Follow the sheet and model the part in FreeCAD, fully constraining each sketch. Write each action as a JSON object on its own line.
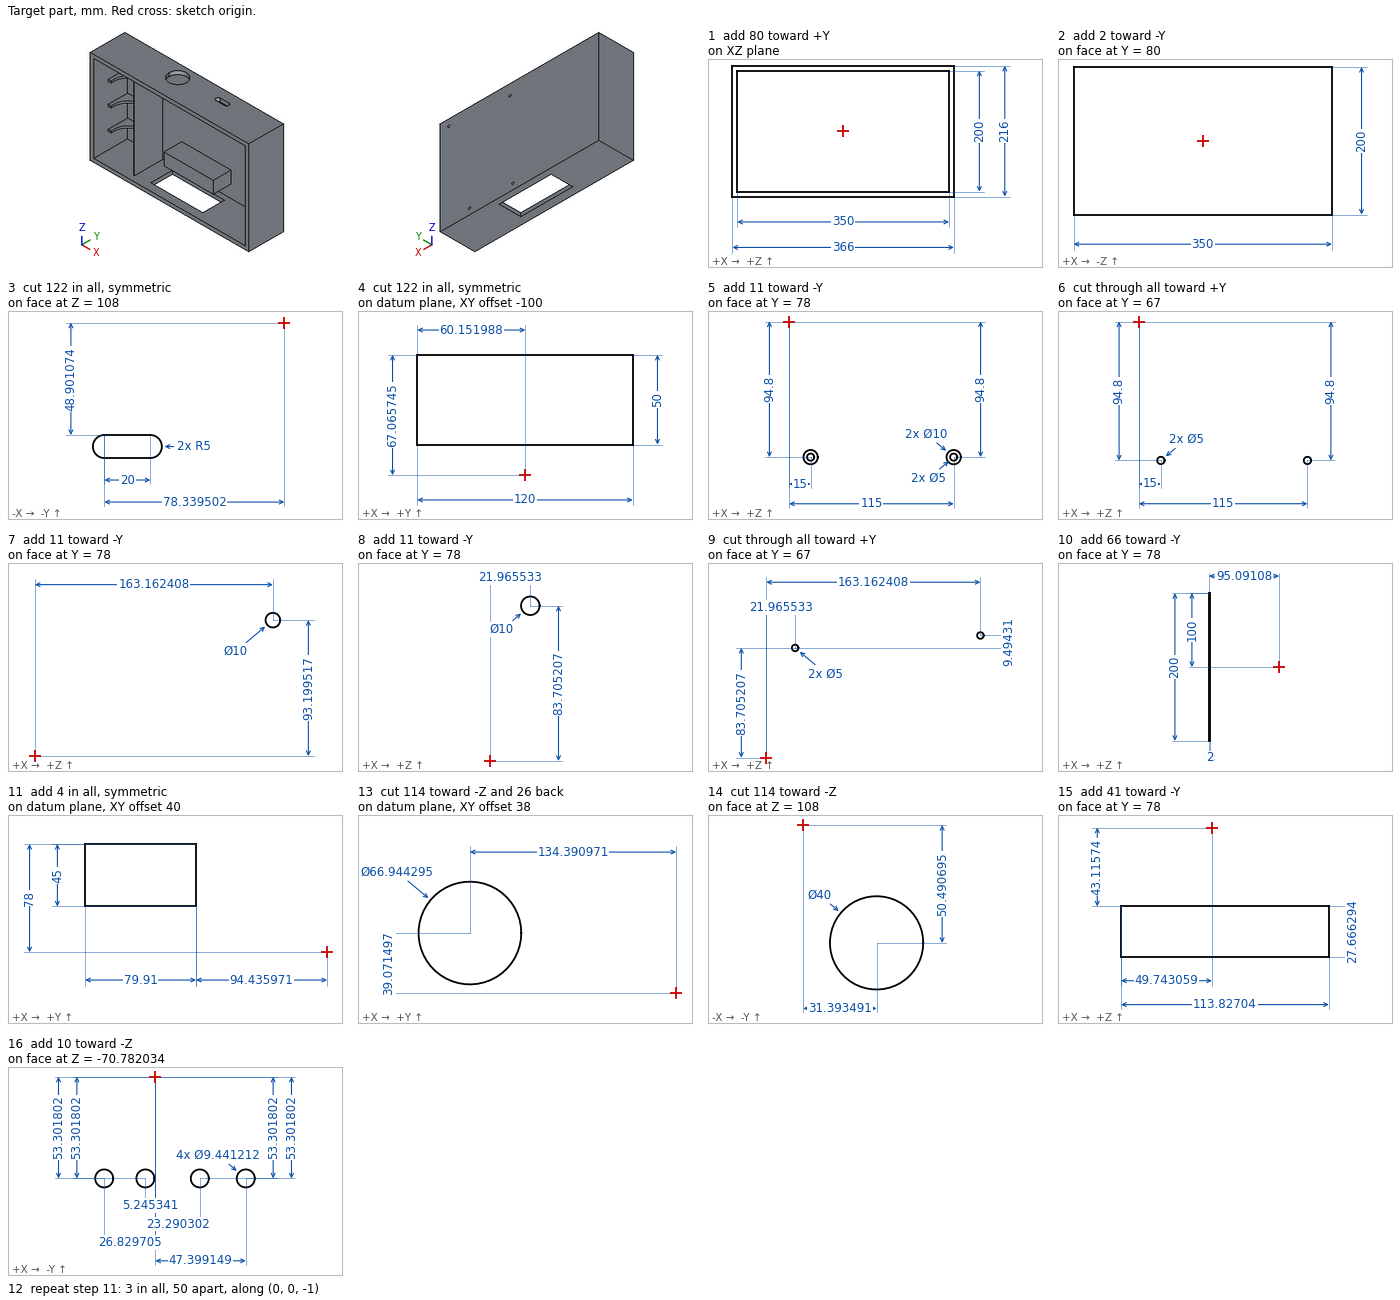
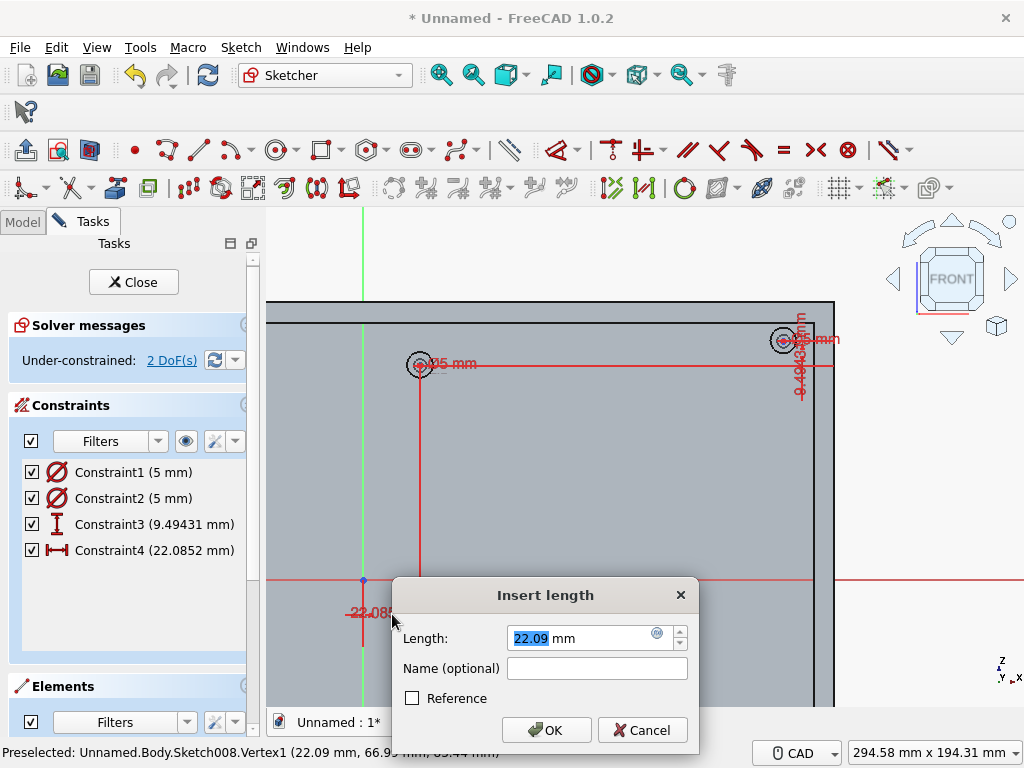
{"action": "type", "text": "21.965533"}
{"action": "key", "text": "Return"}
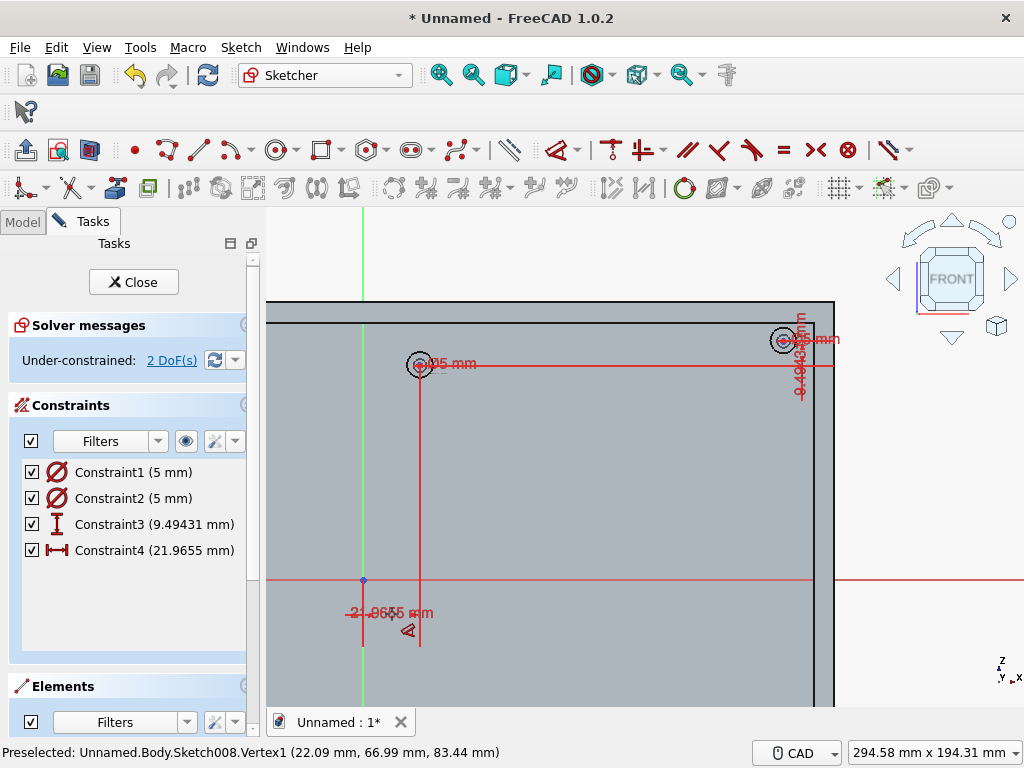
{"action": "left_click", "coordinate": [420, 366]}
{"action": "left_click", "coordinate": [329, 473]}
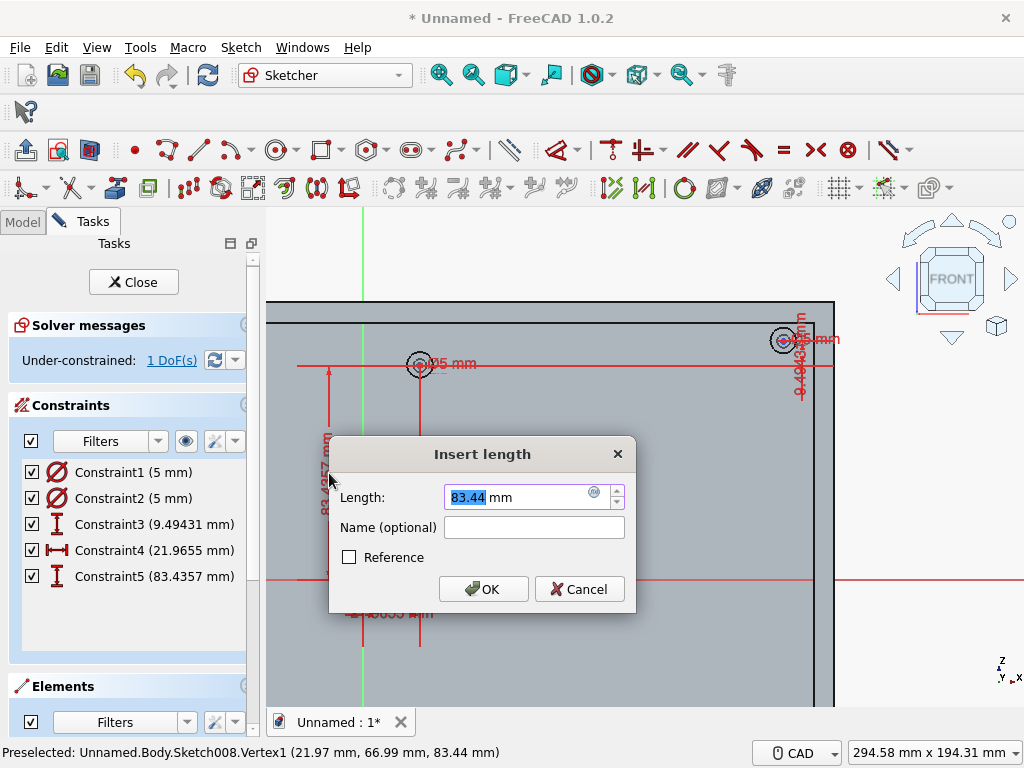
{"action": "type", "text": "83.705207"}
{"action": "key", "text": "Return"}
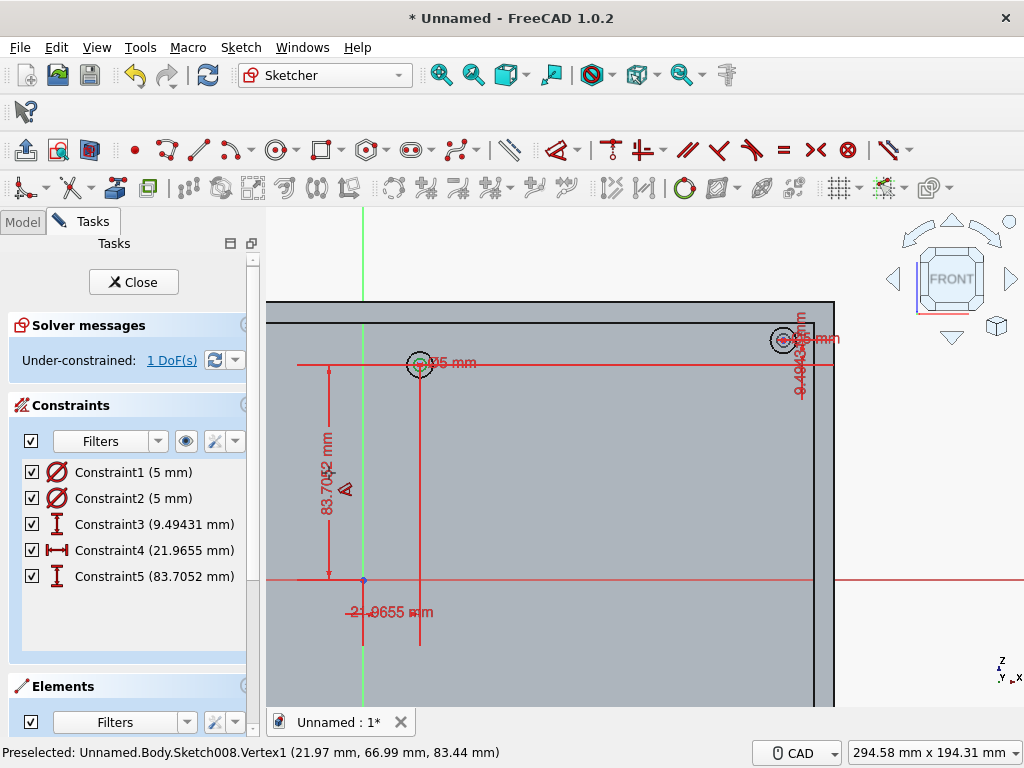
{"action": "left_click", "coordinate": [784, 340]}
{"action": "left_click", "coordinate": [574, 614]}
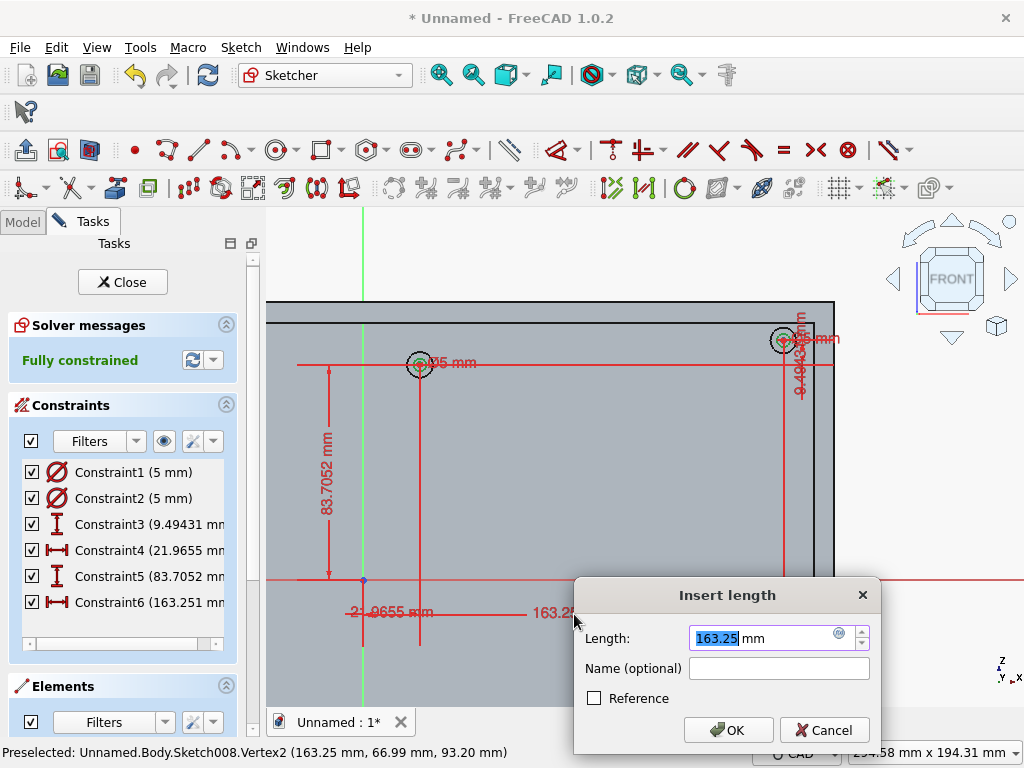
{"action": "type", "text": "163.162408"}
{"action": "key", "text": "Return"}
{"action": "key", "text": "Escape"}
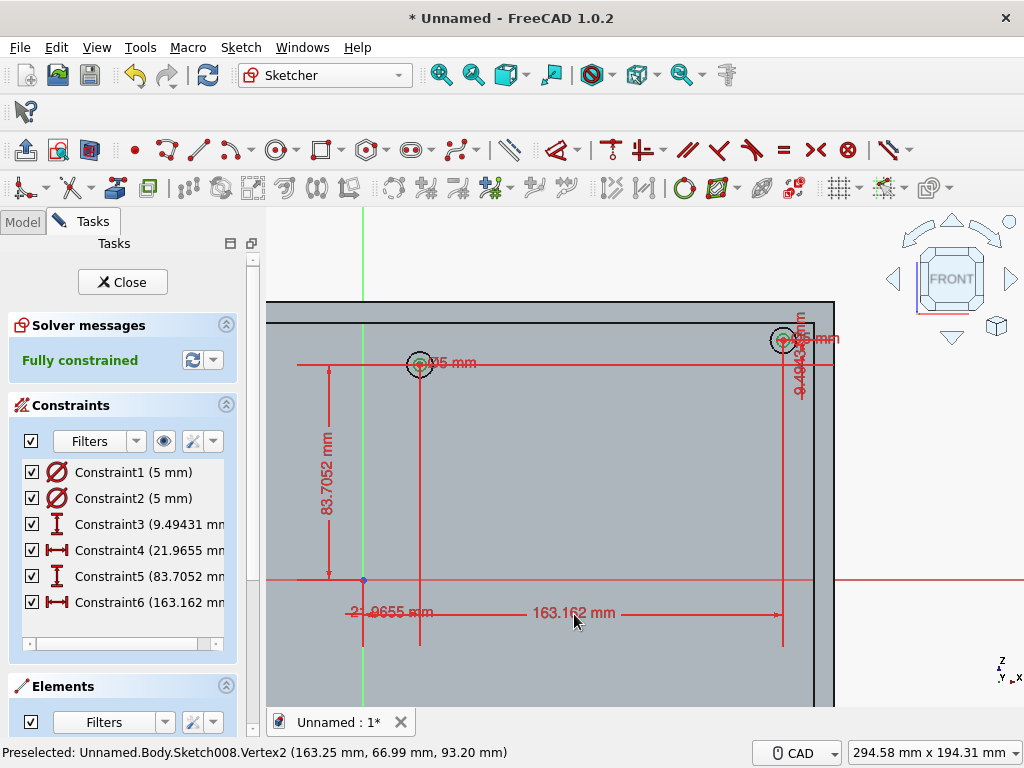
{"action": "left_click", "coordinate": [123, 282]}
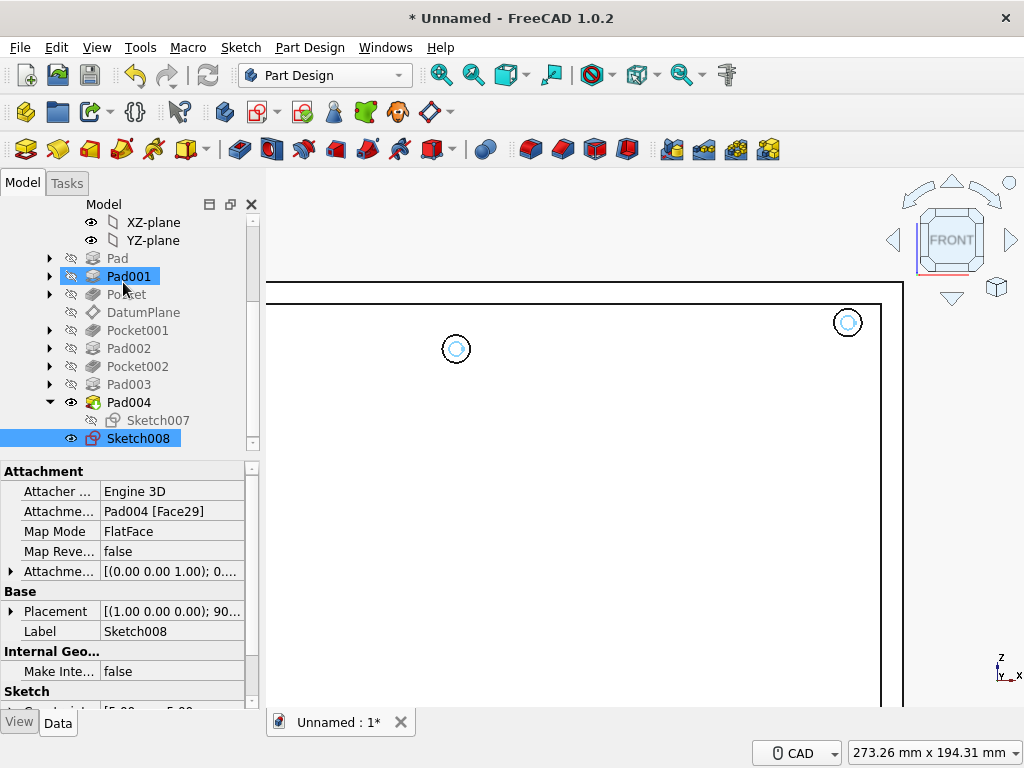
{"action": "left_click", "coordinate": [240, 150]}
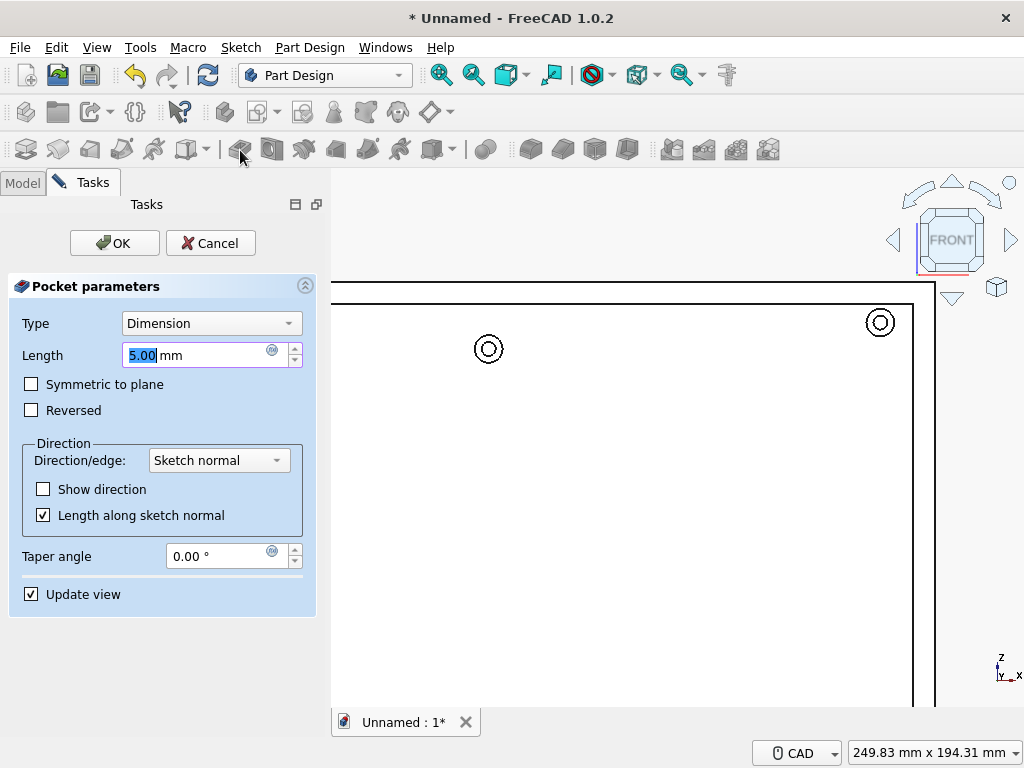
{"action": "left_click", "coordinate": [212, 324]}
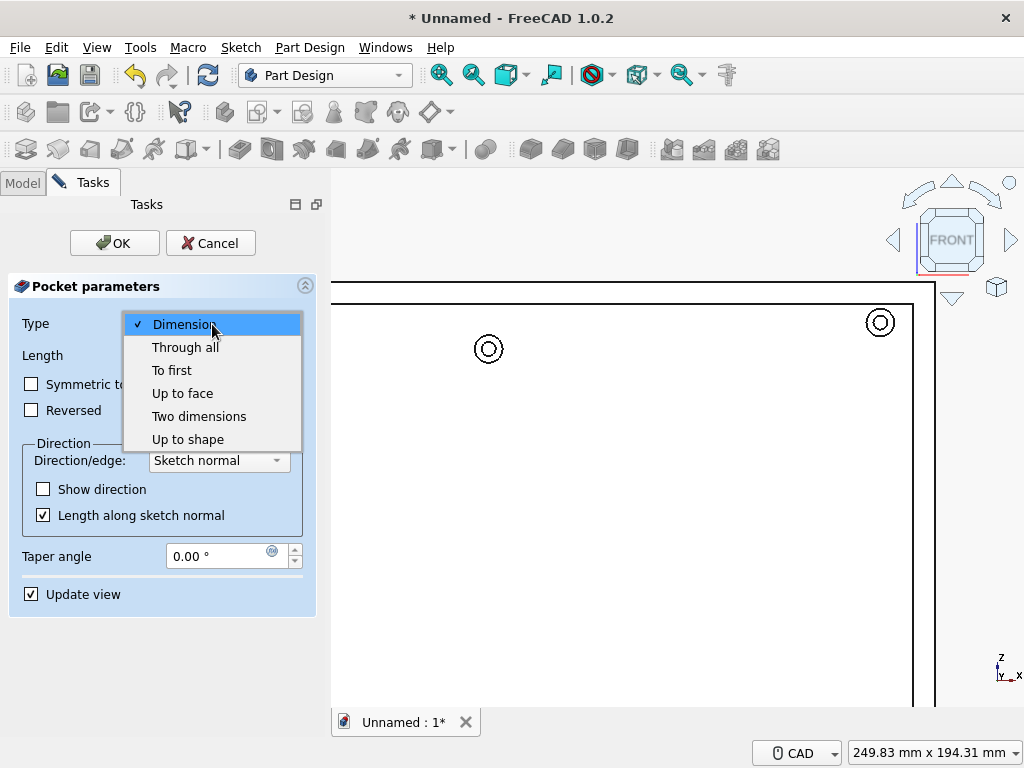
{"action": "left_click", "coordinate": [212, 348]}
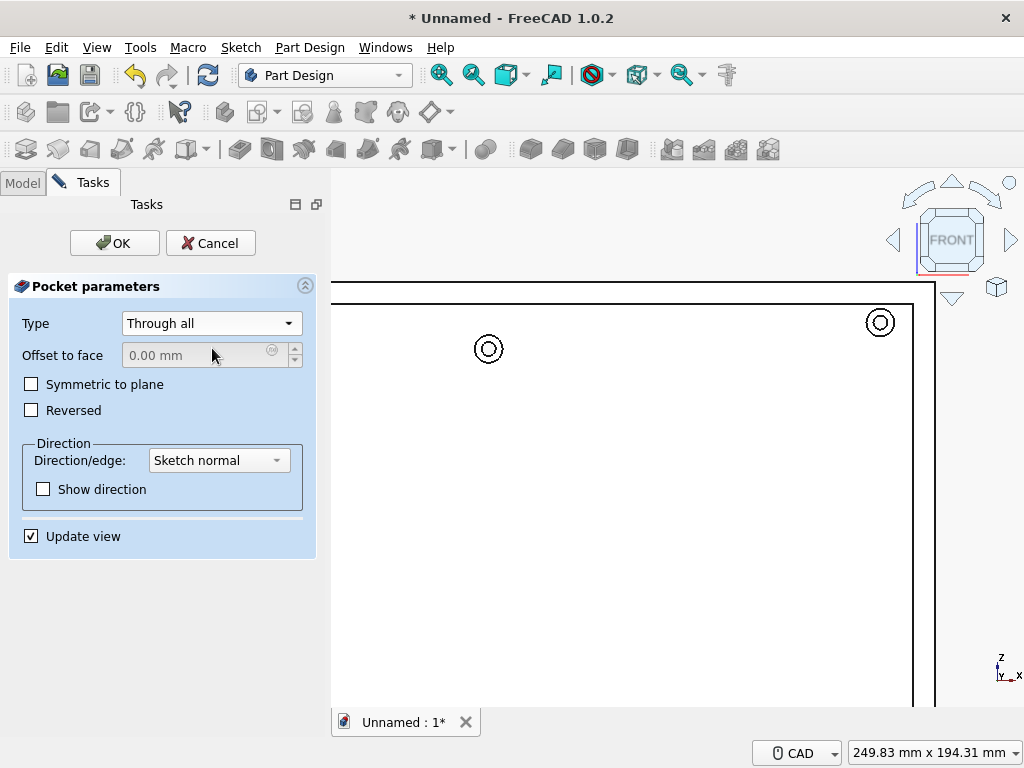
{"action": "left_click", "coordinate": [115, 243]}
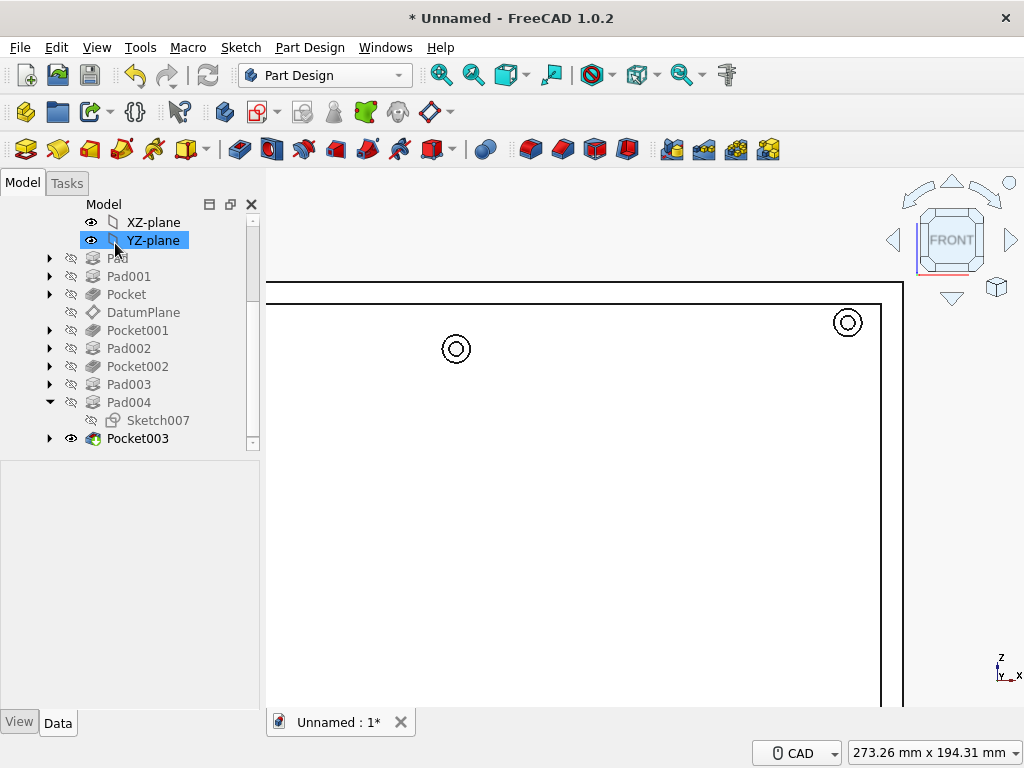
{"action": "left_click", "coordinate": [442, 76]}